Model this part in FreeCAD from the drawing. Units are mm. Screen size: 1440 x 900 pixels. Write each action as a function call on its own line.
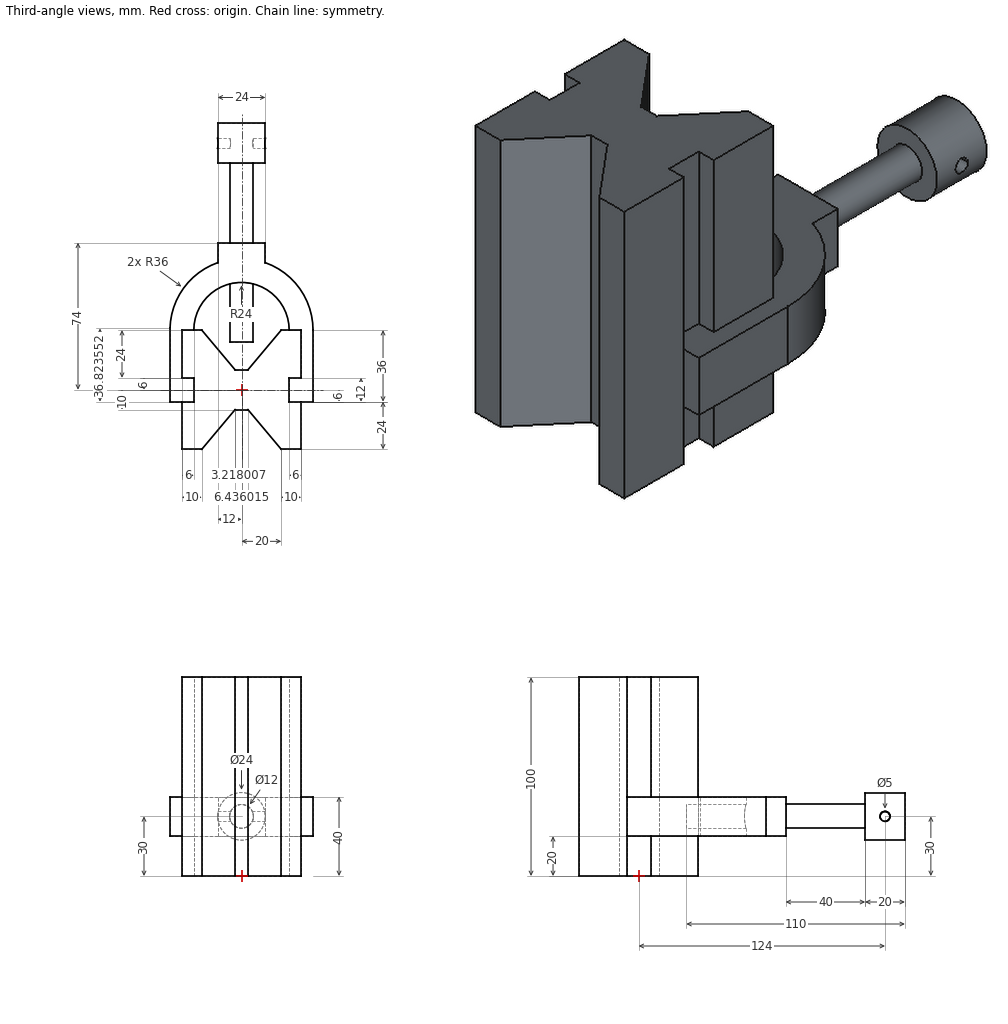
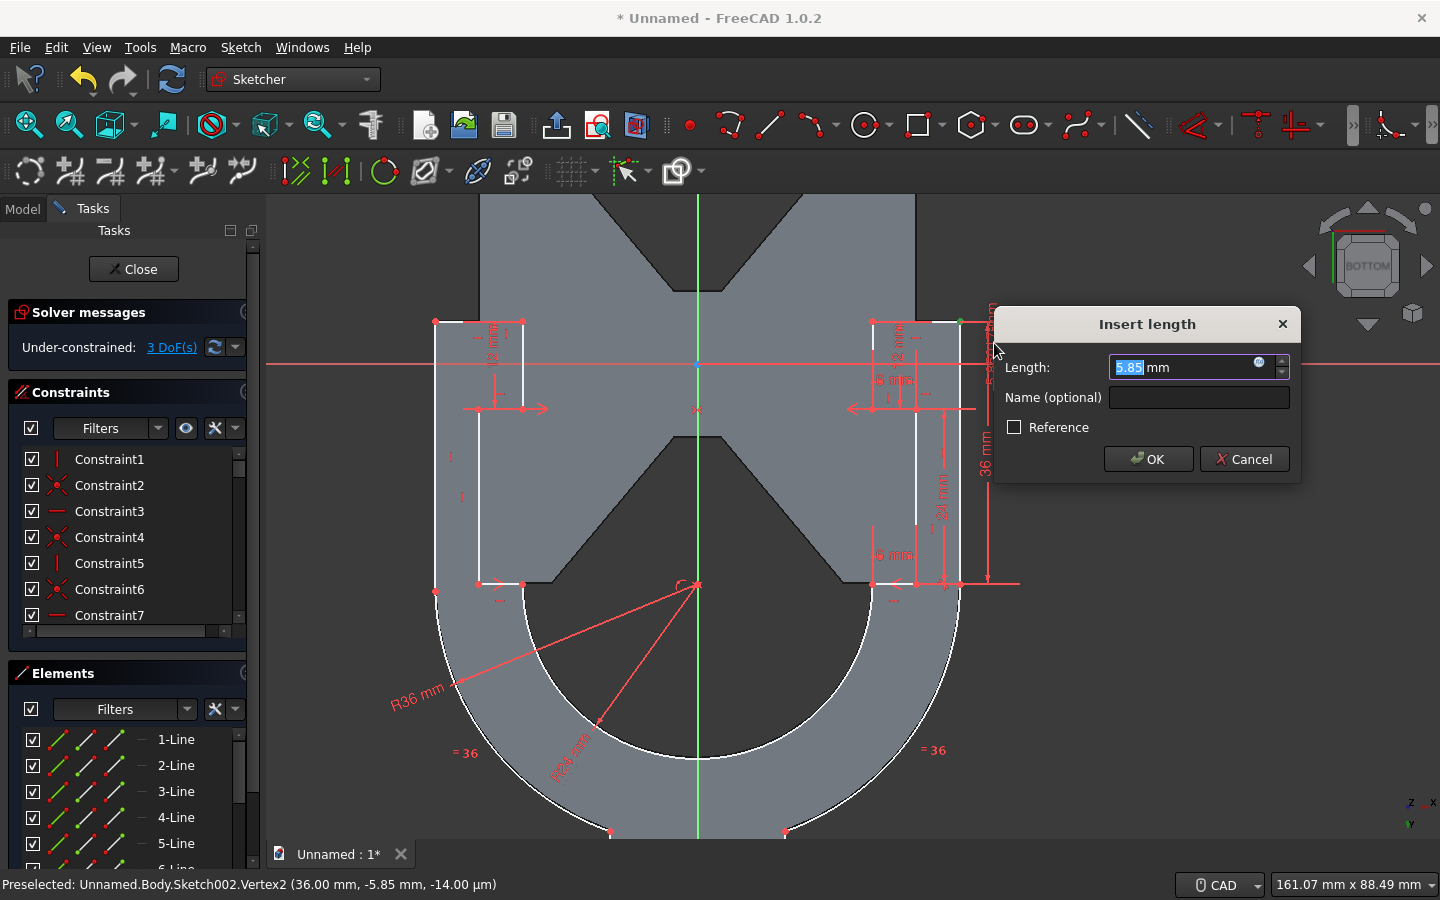
text(6)
key(Return)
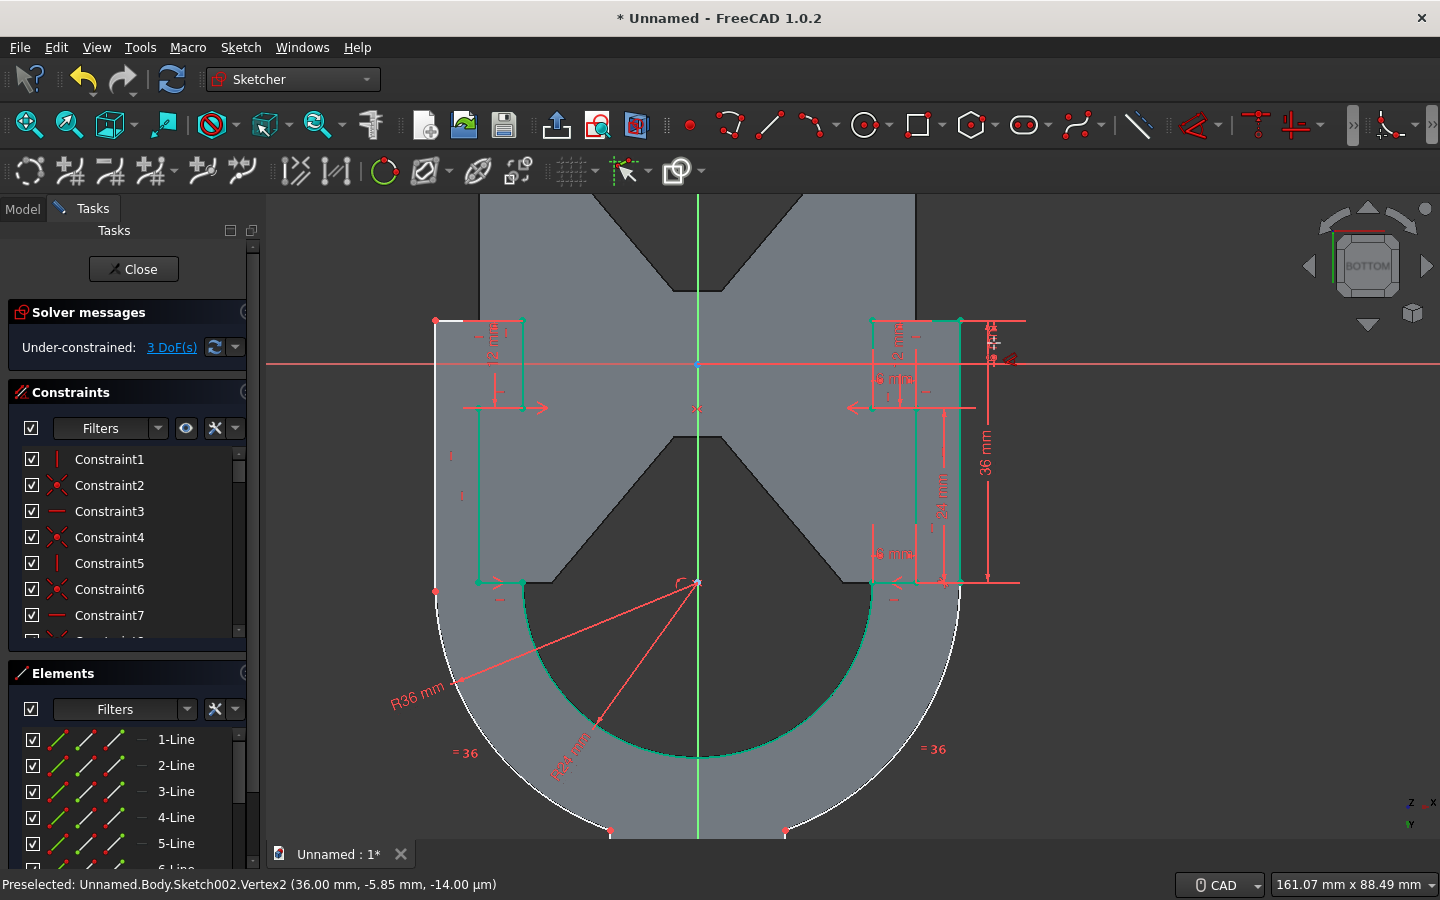
scroll(961, 322, down, 2)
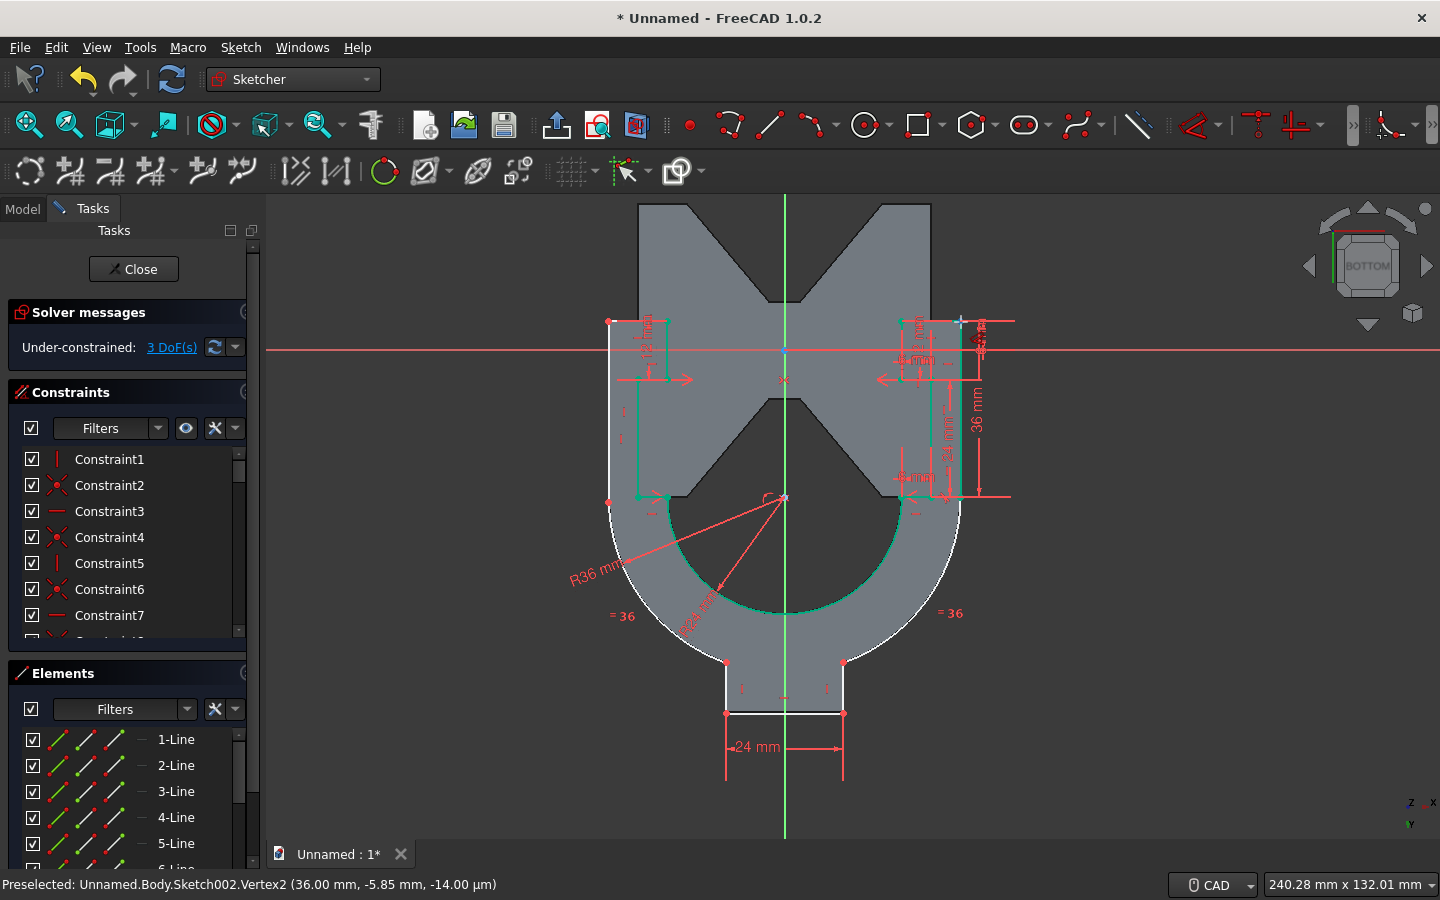
click(726, 663)
click(755, 316)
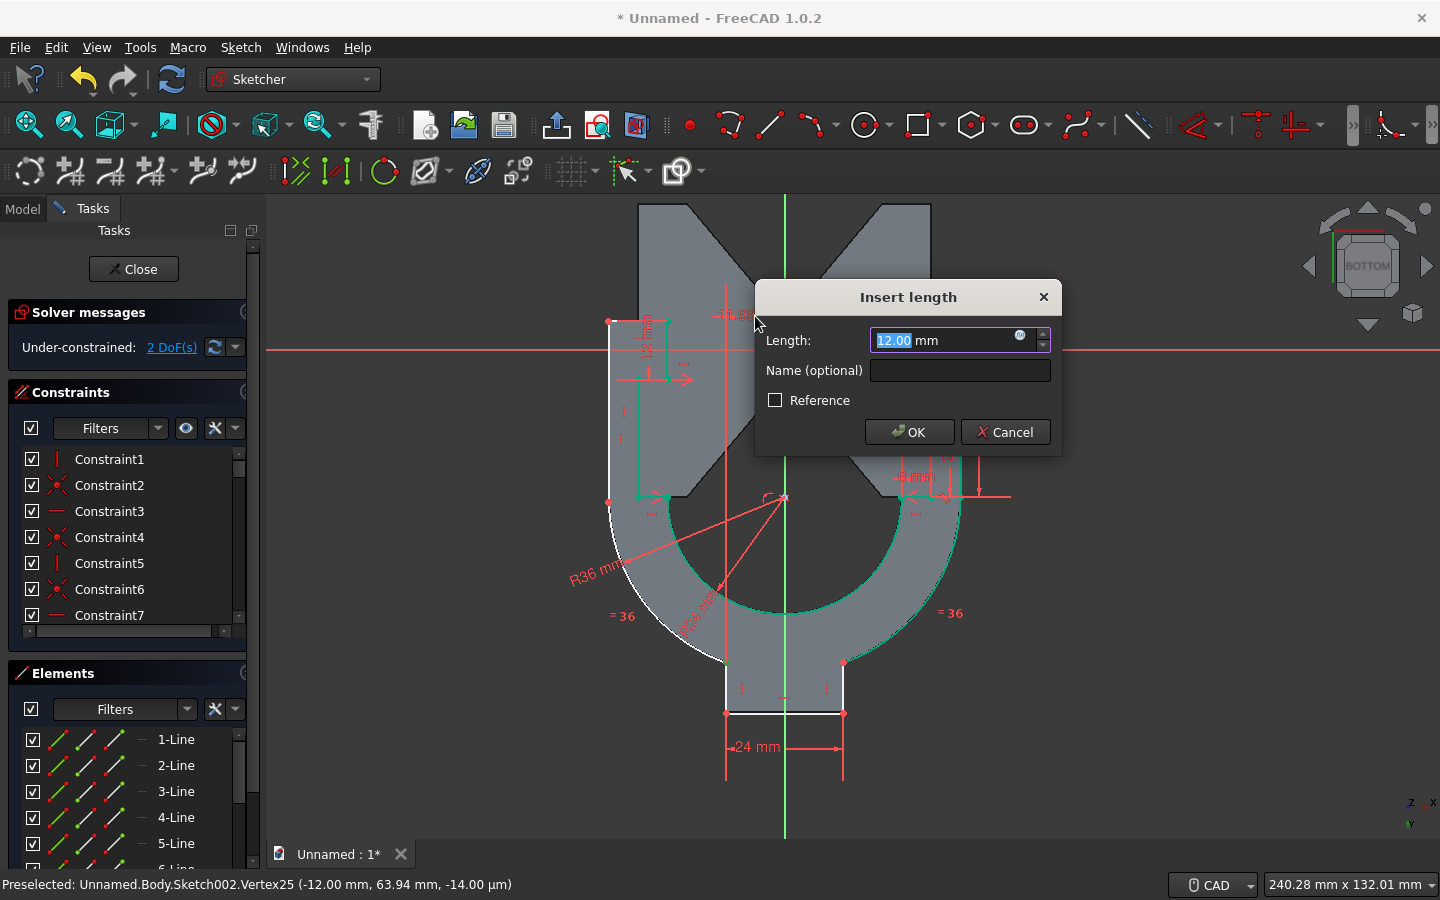
text(12)
key(Return)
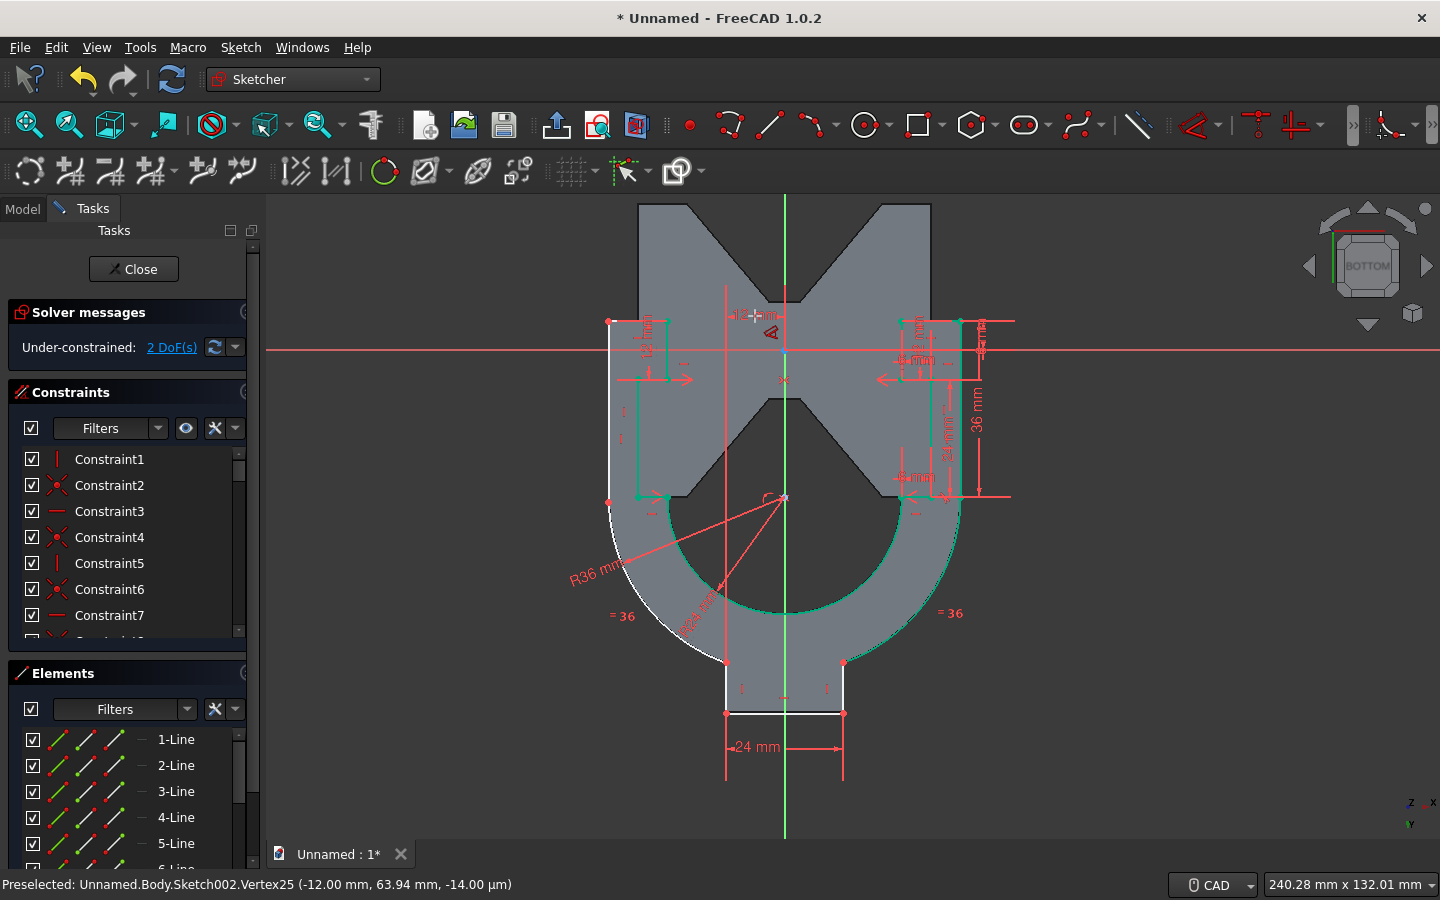
click(726, 714)
click(692, 532)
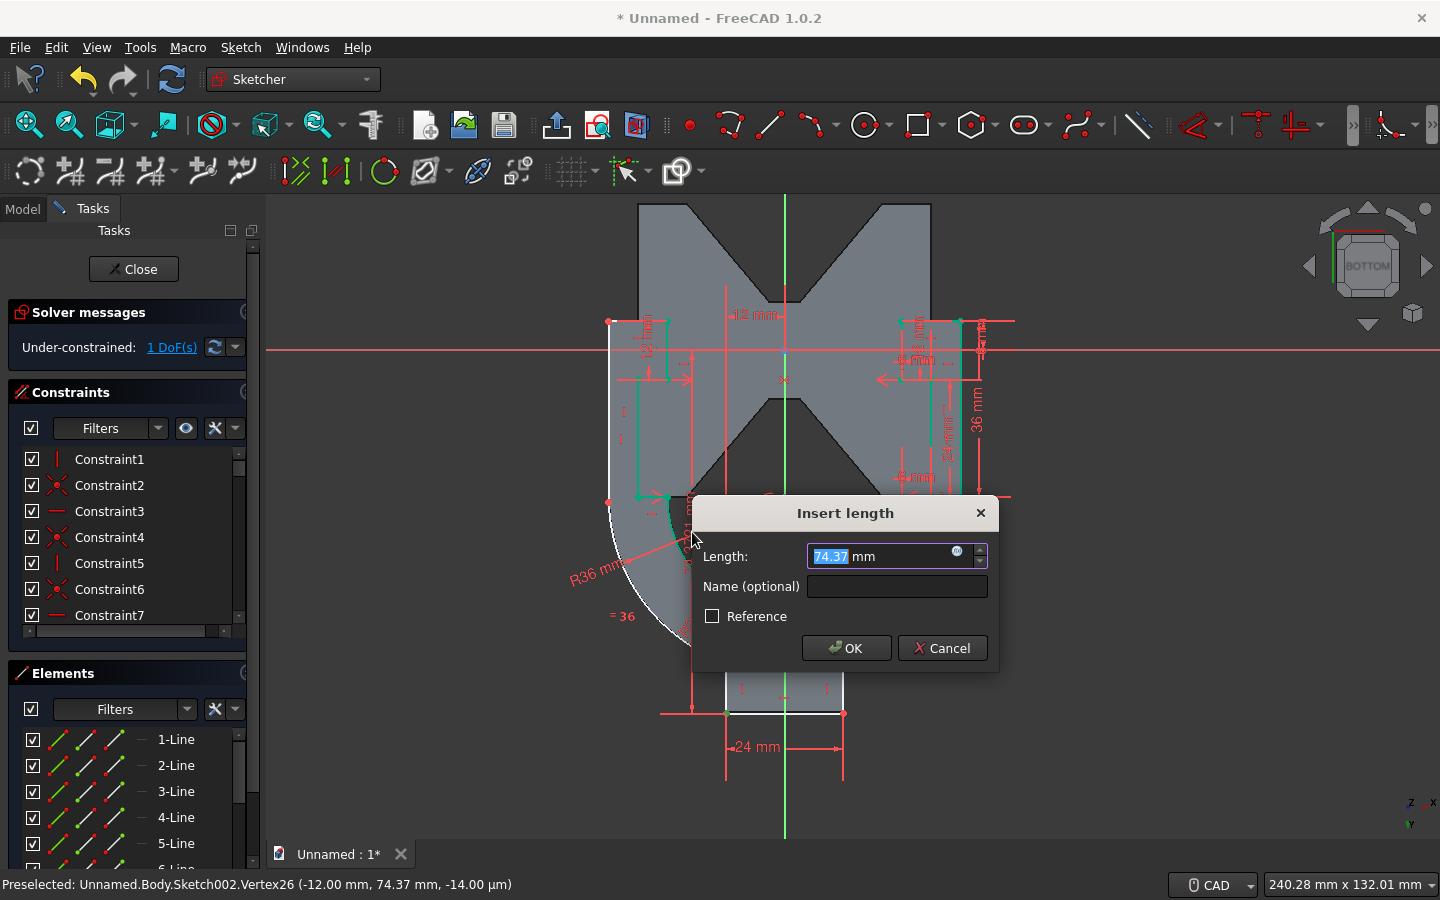
text(74)
key(Return)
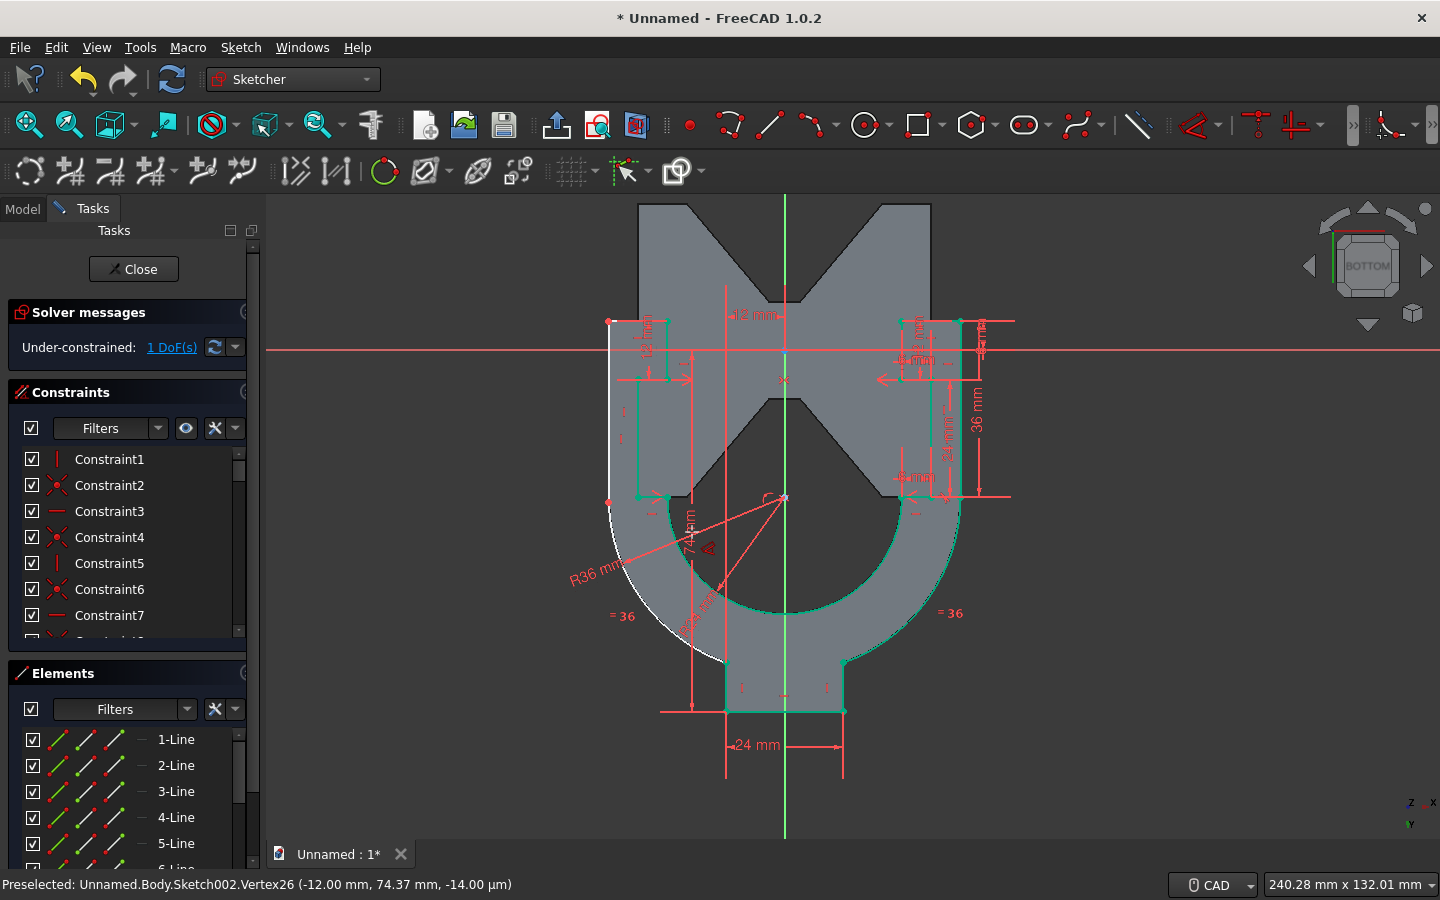
click(609, 376)
click(575, 412)